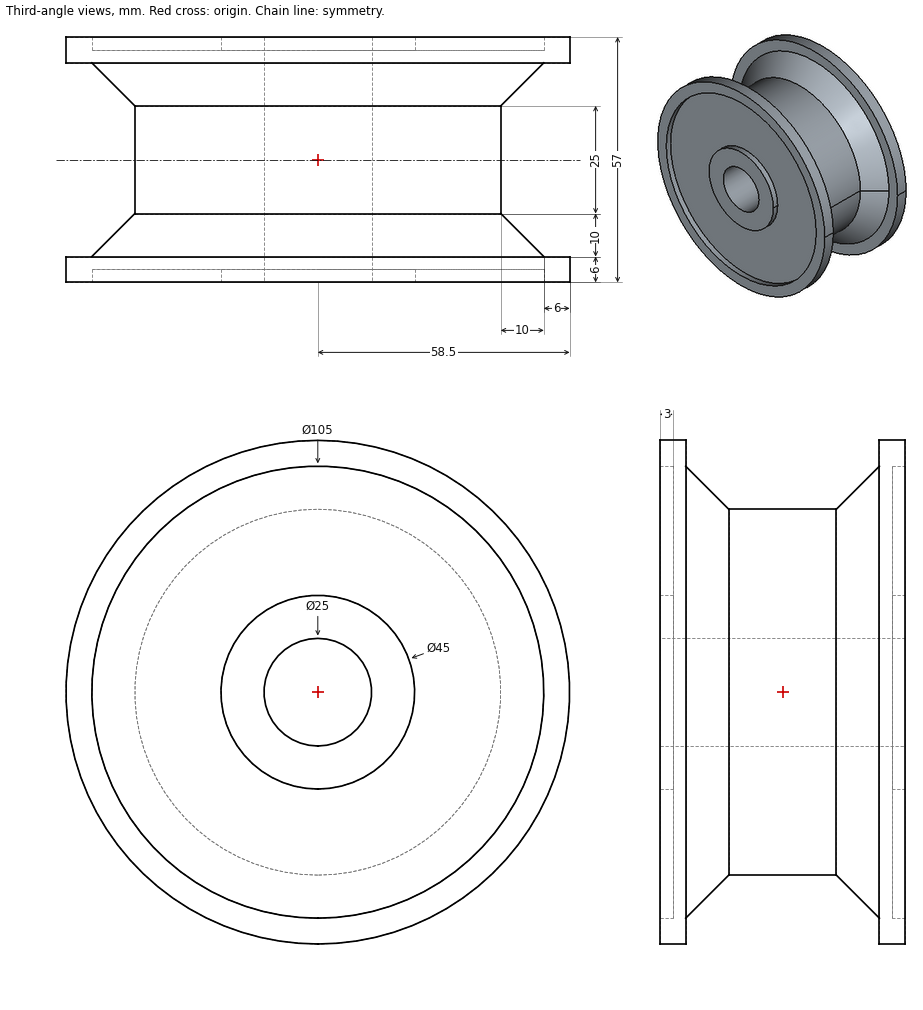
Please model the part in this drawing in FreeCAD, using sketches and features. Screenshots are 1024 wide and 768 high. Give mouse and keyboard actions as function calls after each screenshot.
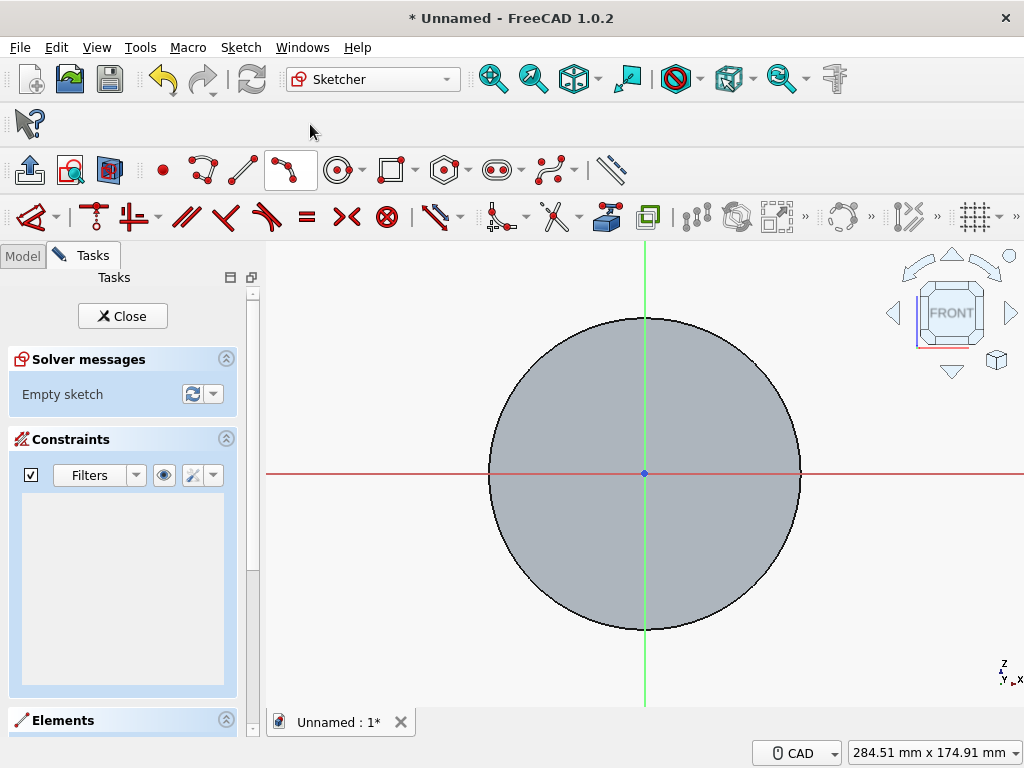
scroll(667, 474, up, 7)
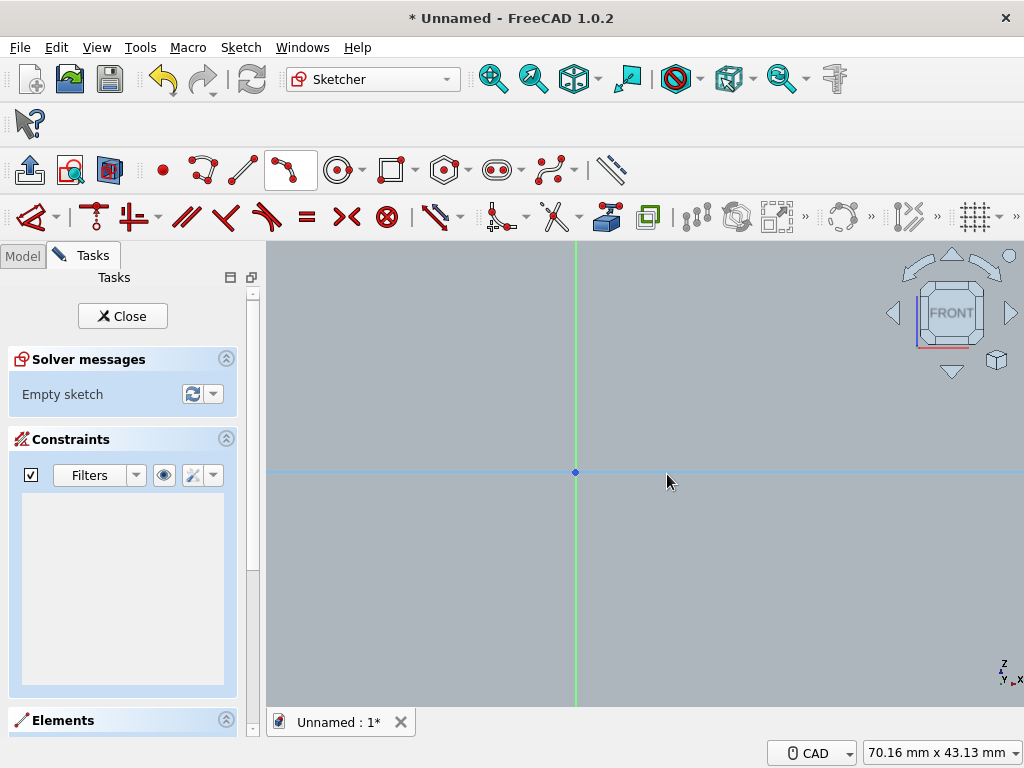
click(338, 170)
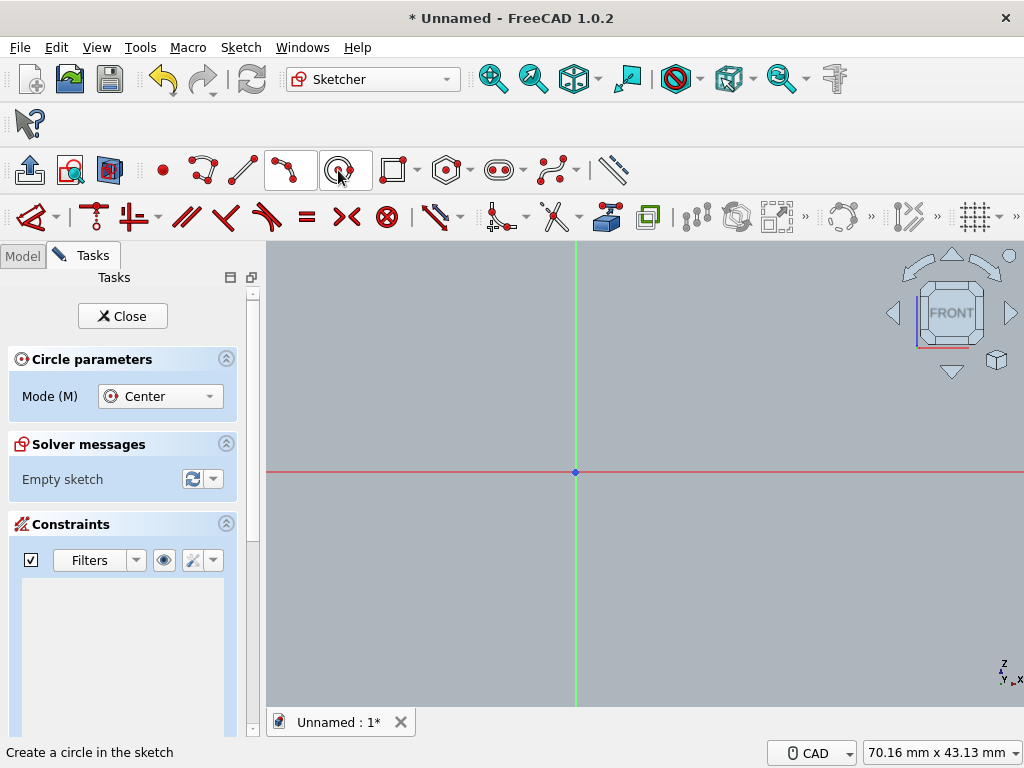
click(576, 472)
click(671, 377)
key(Escape)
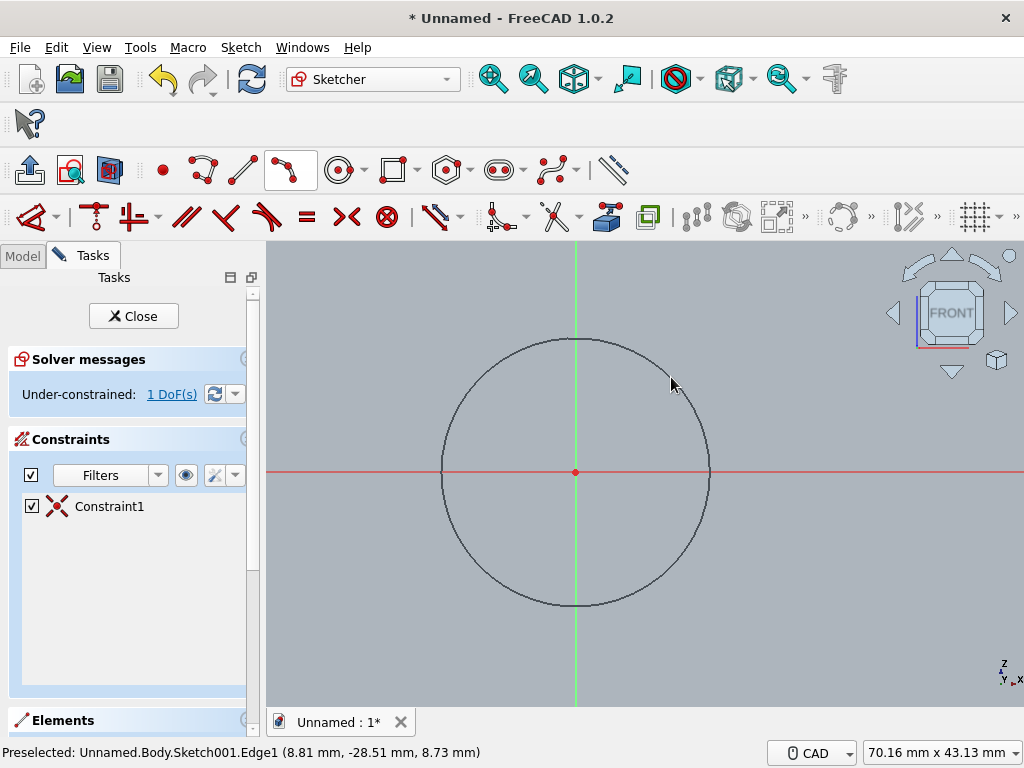
click(32, 218)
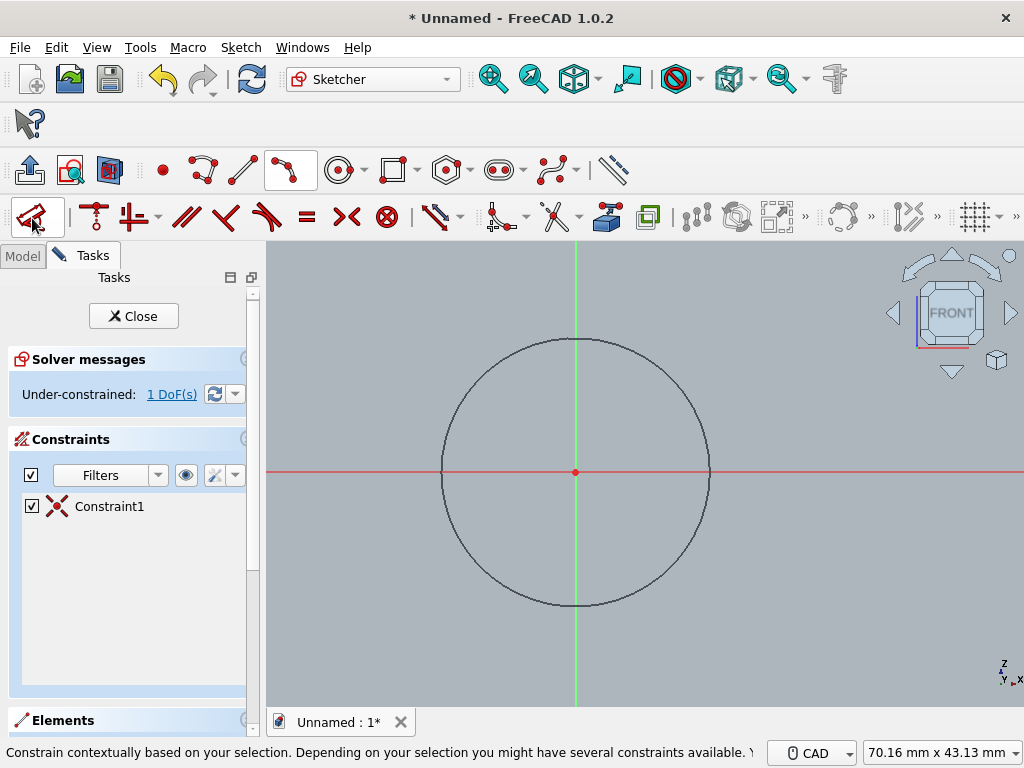
click(670, 377)
click(692, 354)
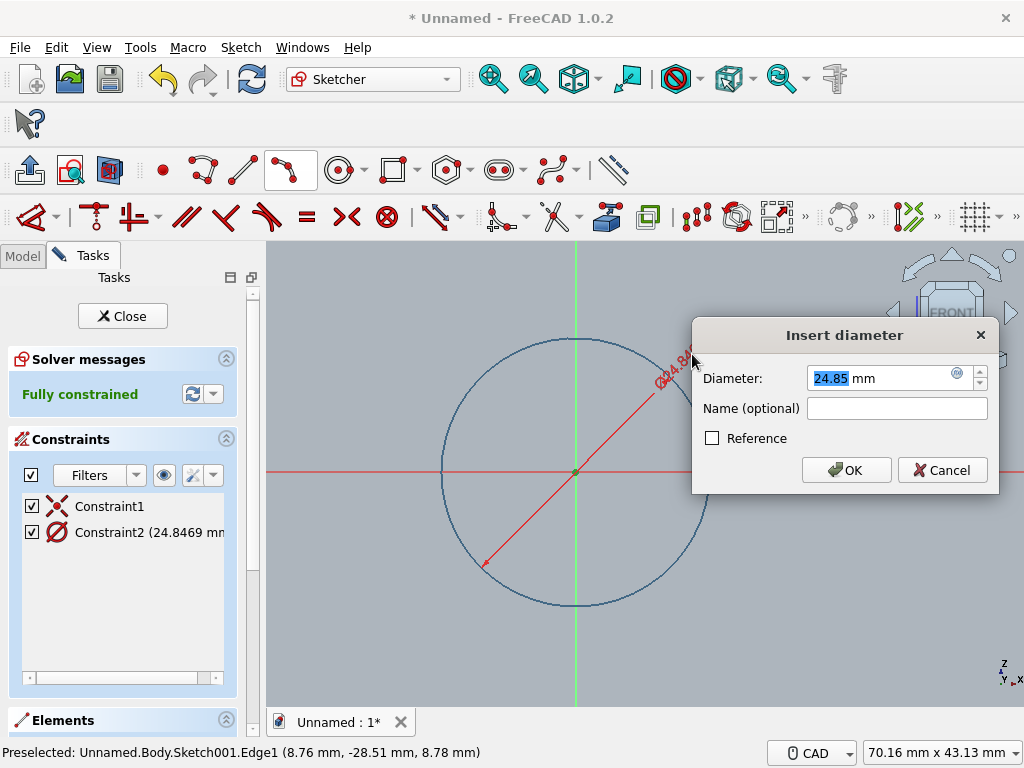
text(25)
key(Return)
key(Escape)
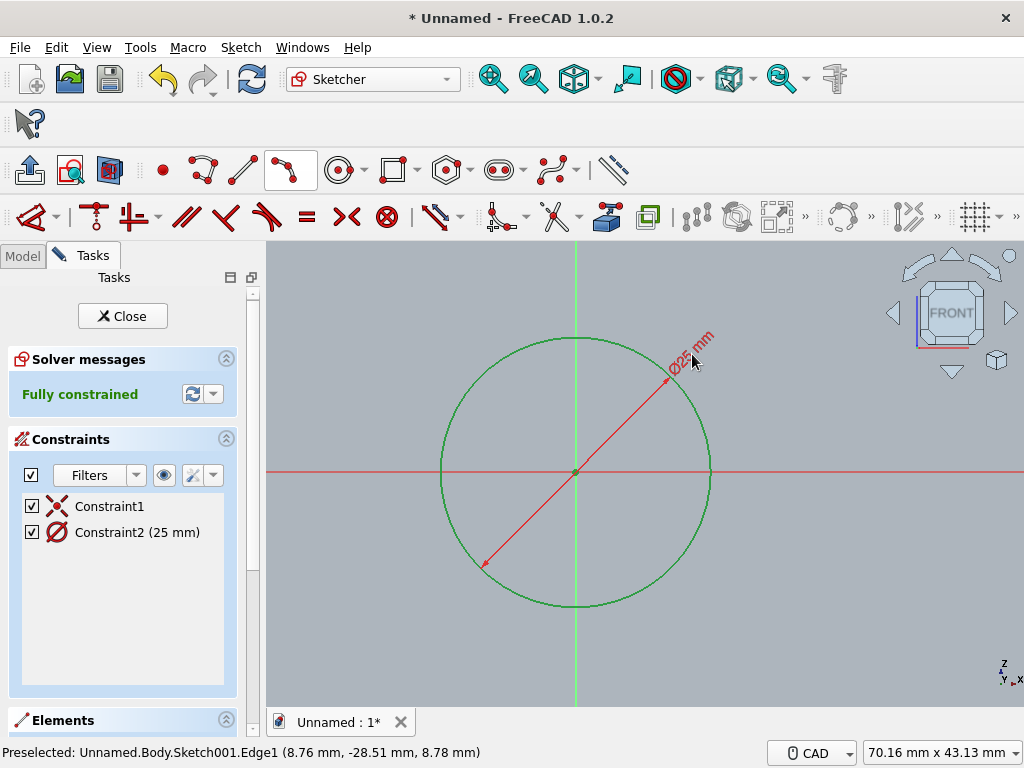
click(123, 316)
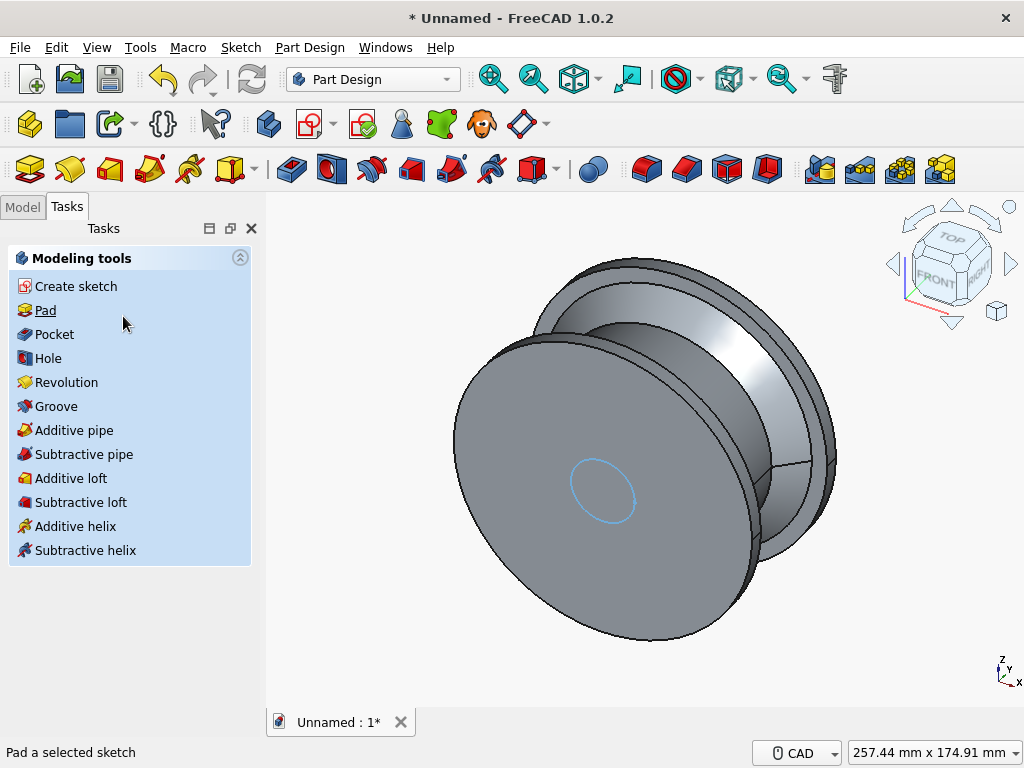
click(292, 170)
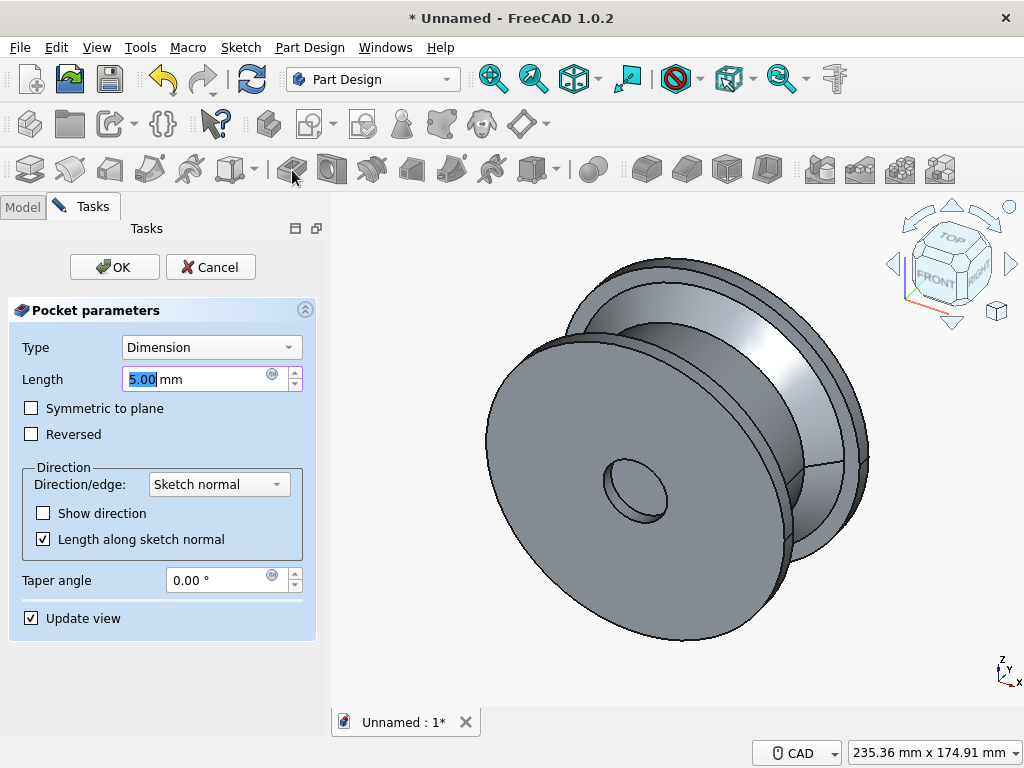
click(212, 348)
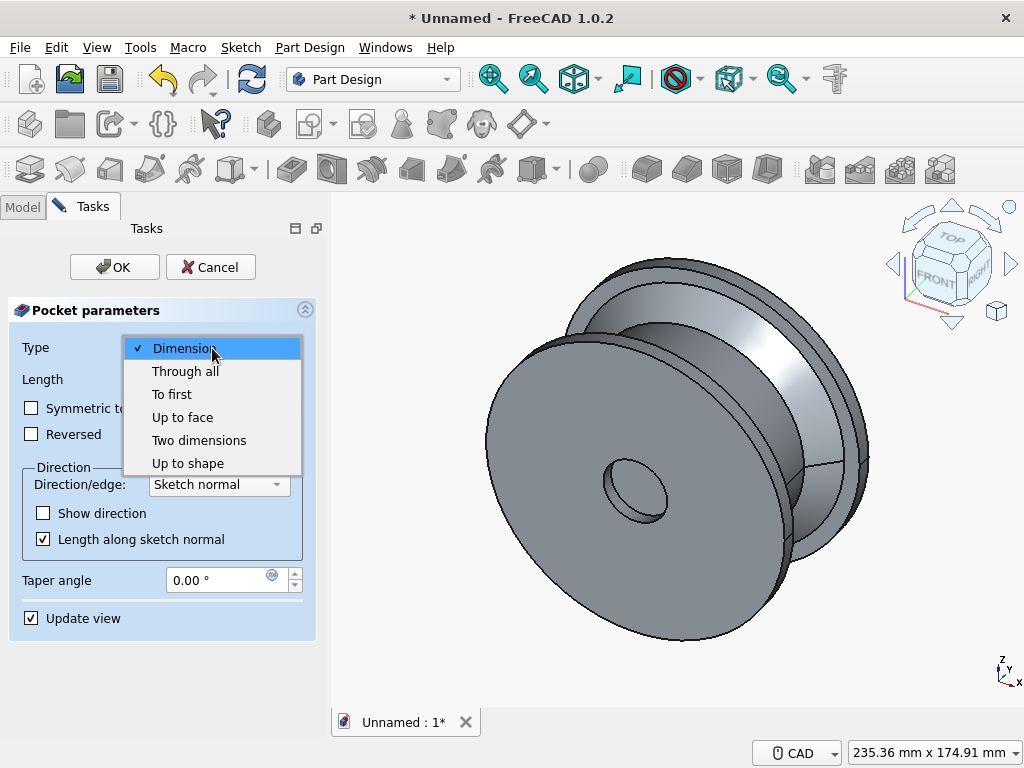
click(212, 372)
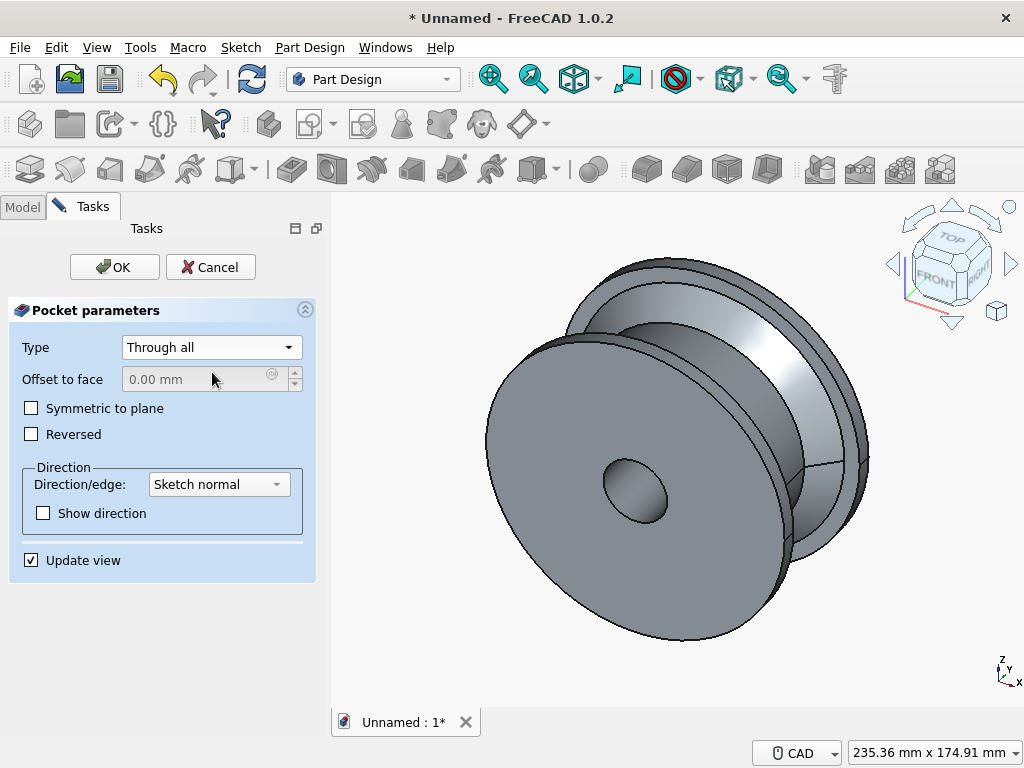
click(115, 267)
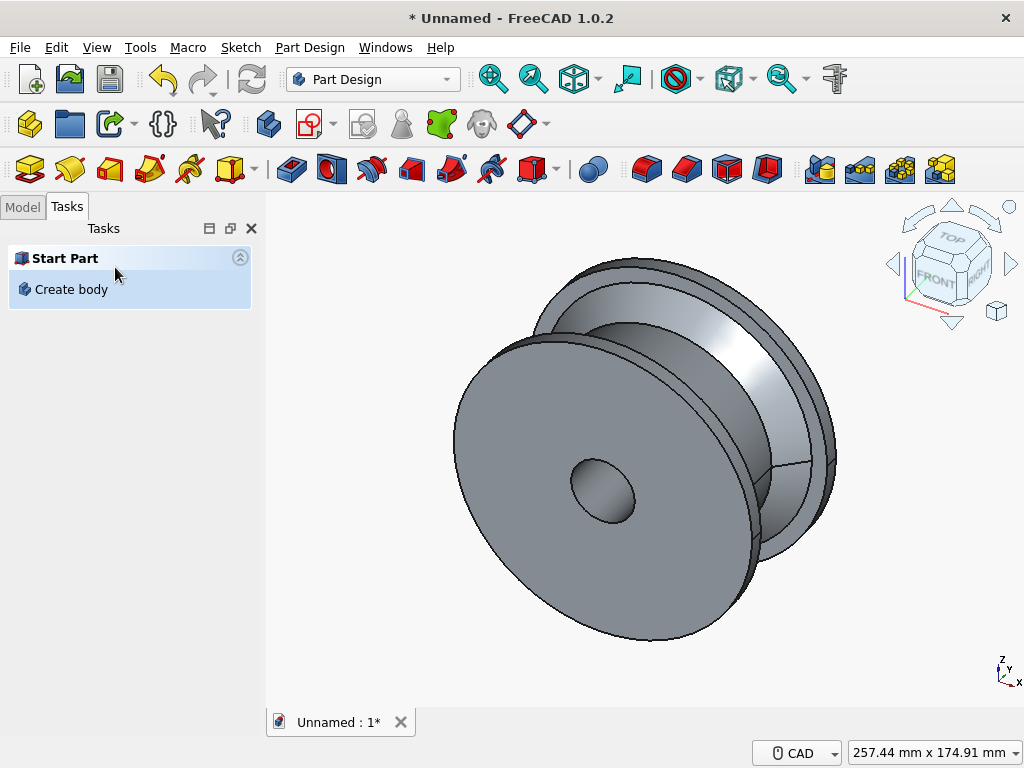
click(688, 478)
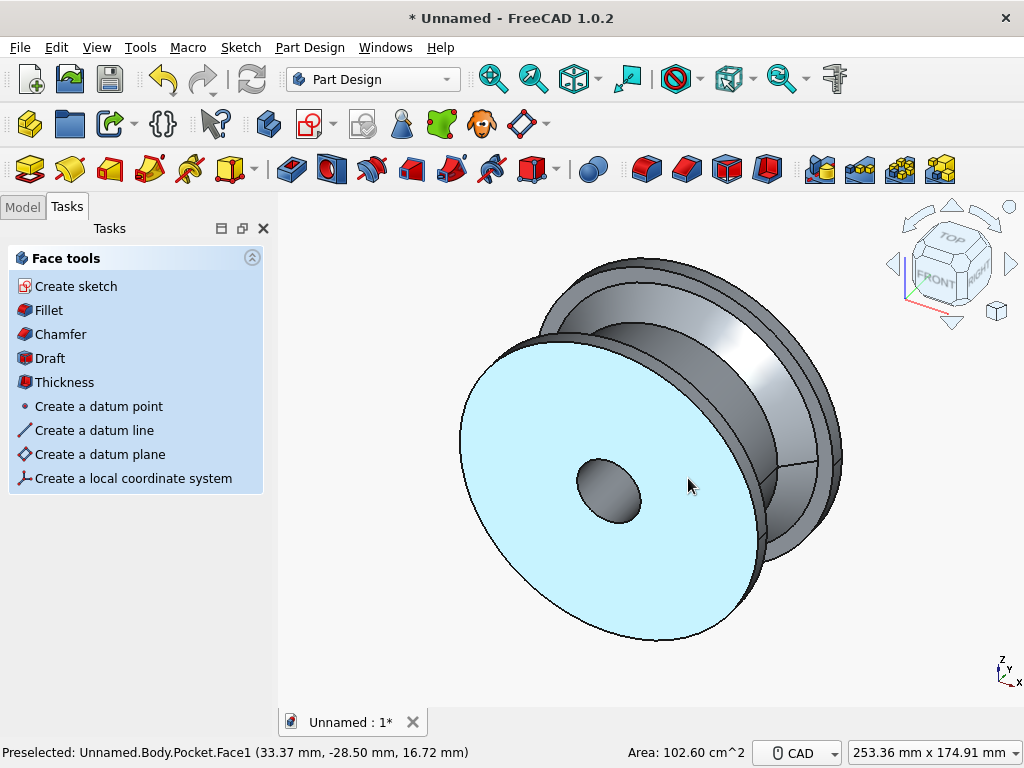
click(310, 124)